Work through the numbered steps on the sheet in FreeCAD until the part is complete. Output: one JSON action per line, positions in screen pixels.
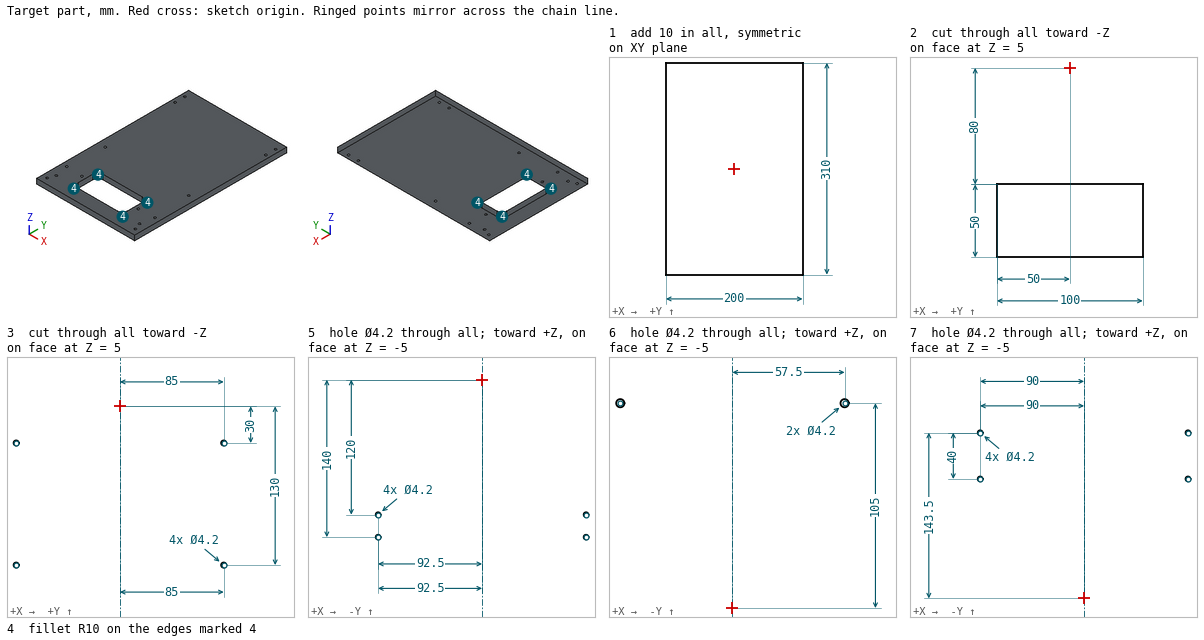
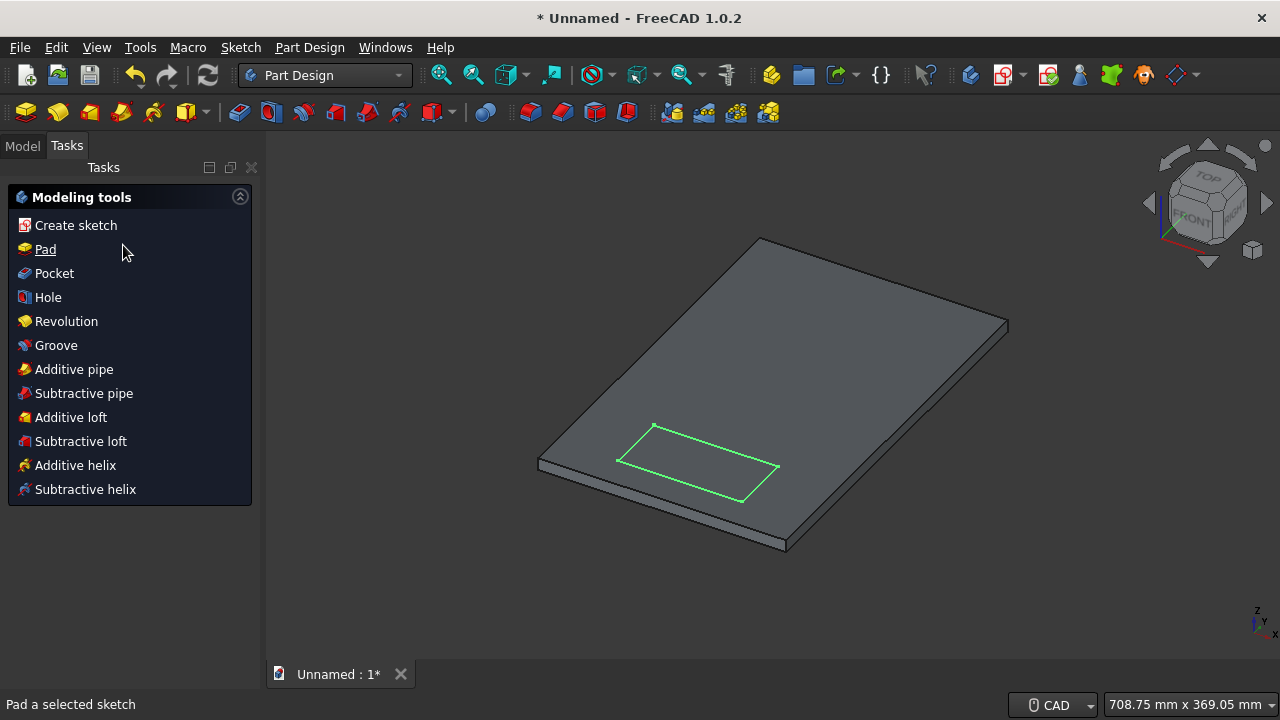
{"action": "left_click", "coordinate": [240, 112]}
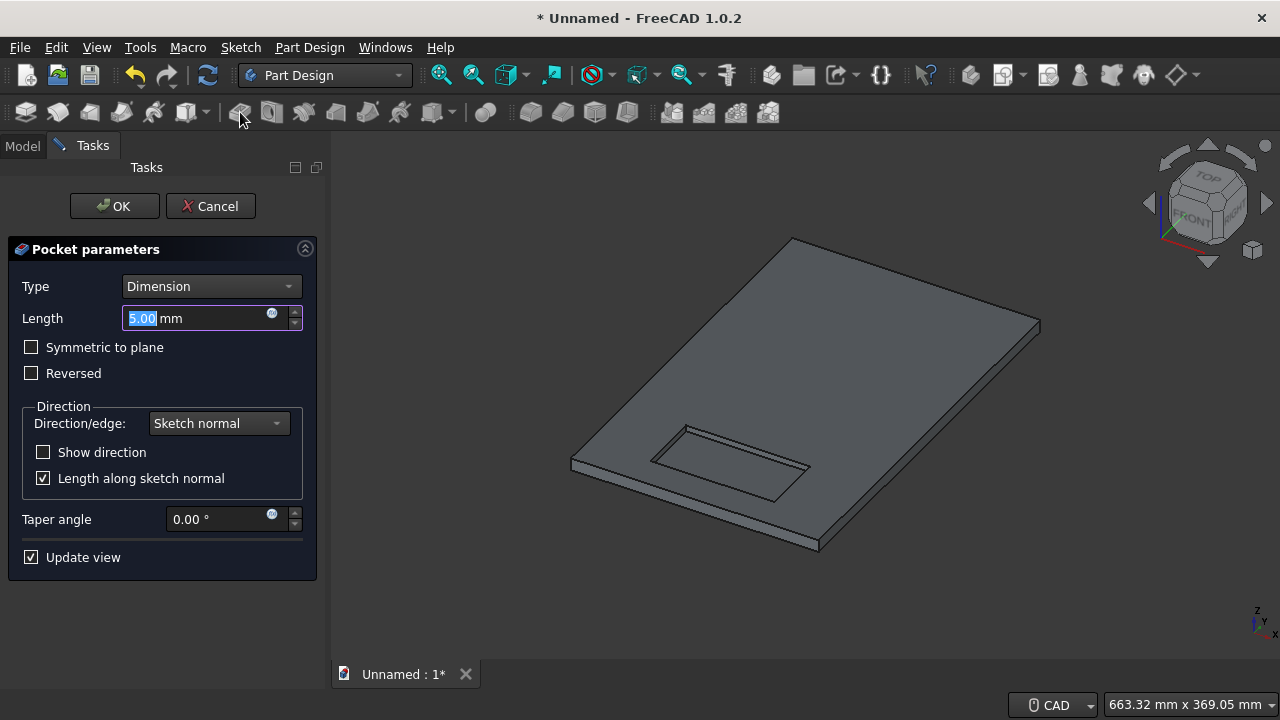
{"action": "left_click", "coordinate": [212, 286]}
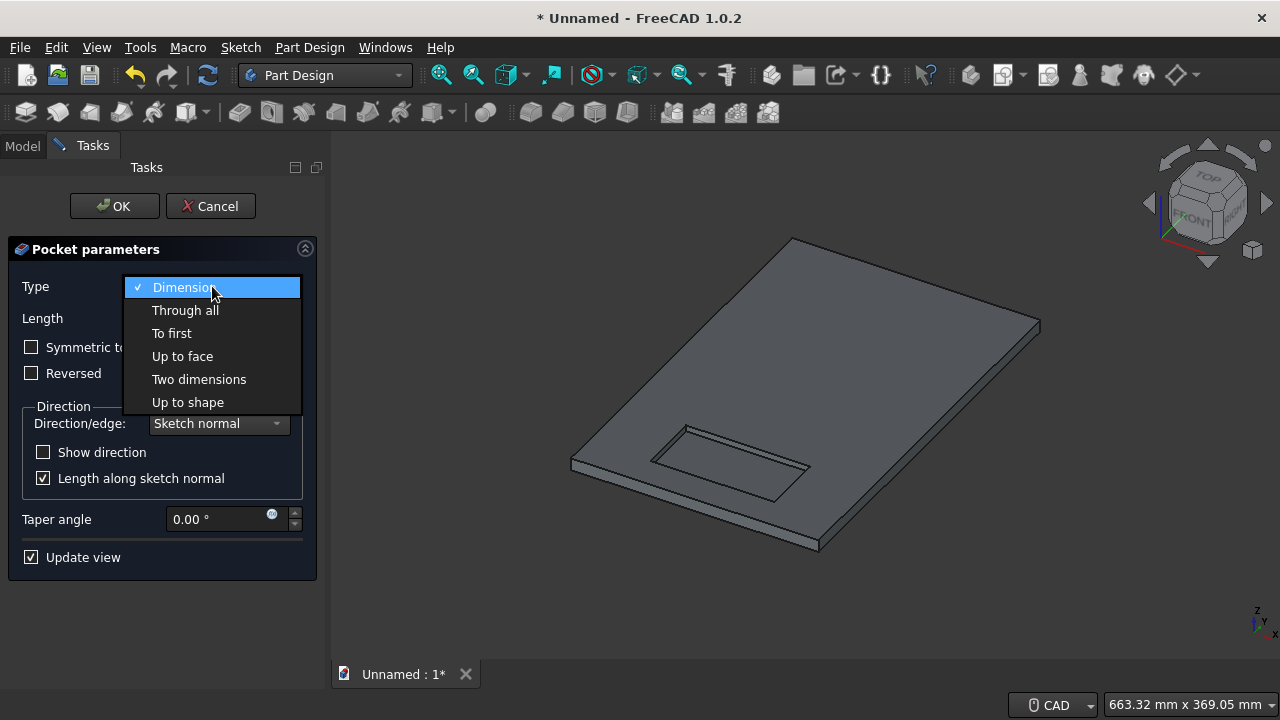
{"action": "left_click", "coordinate": [212, 310]}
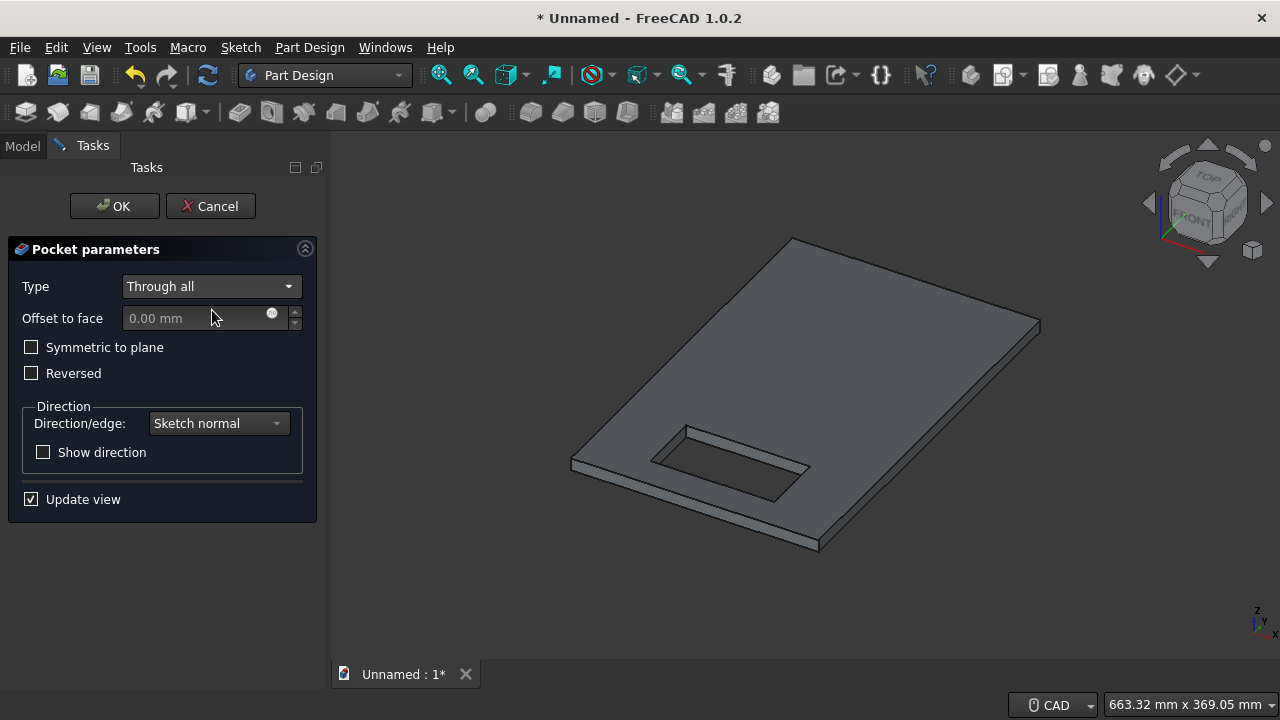
{"action": "left_click", "coordinate": [115, 206]}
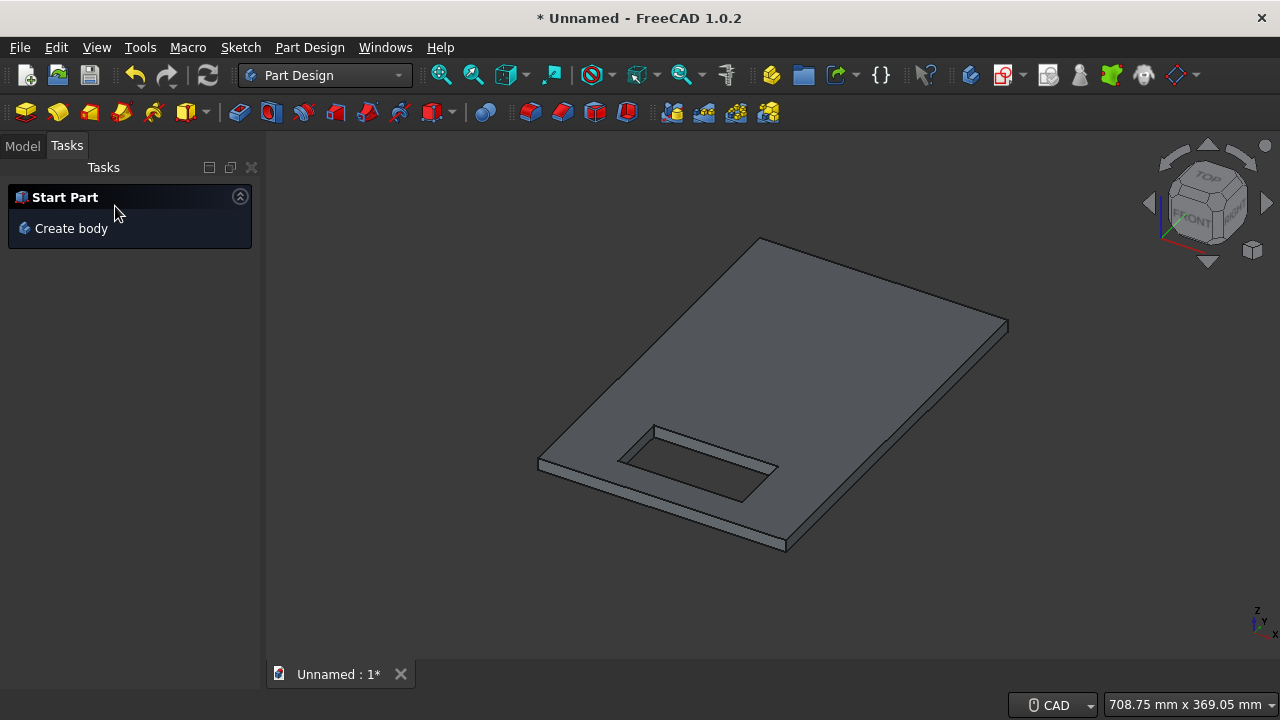
{"action": "left_click", "coordinate": [805, 357]}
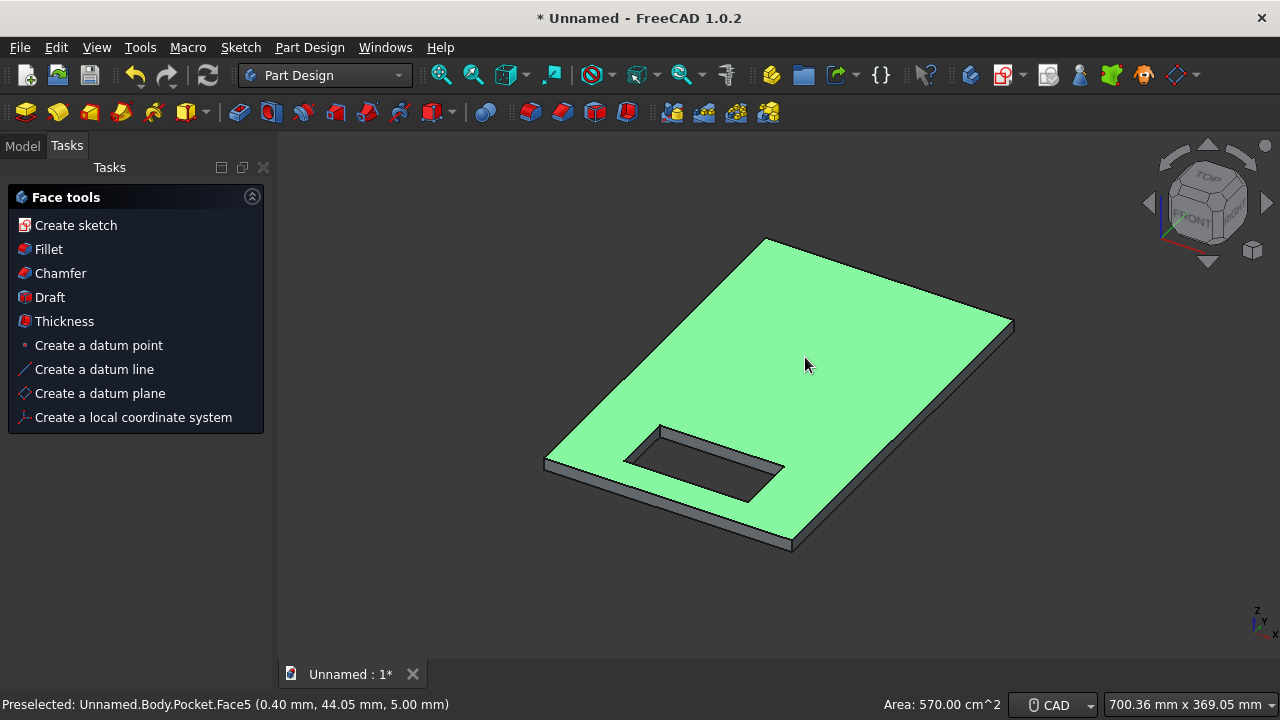
{"action": "left_click", "coordinate": [1004, 76]}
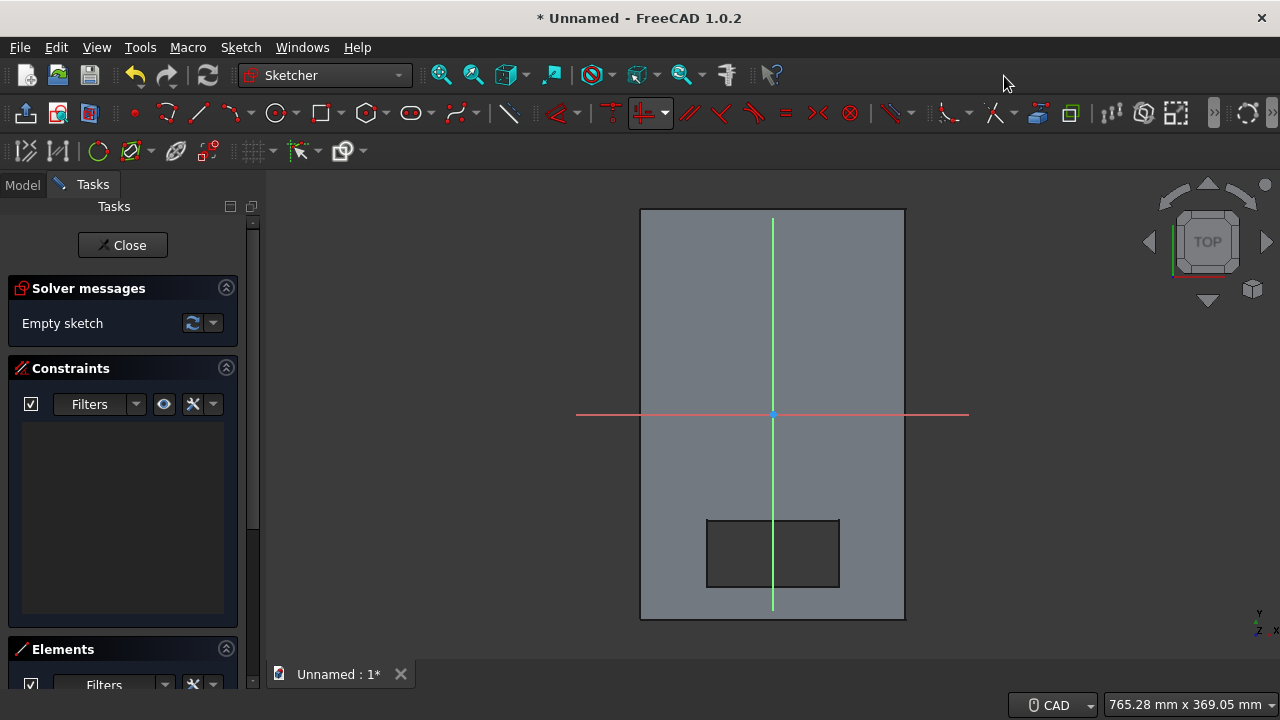
{"action": "scroll", "coordinate": [856, 608], "scroll_direction": "up", "scroll_amount": 3}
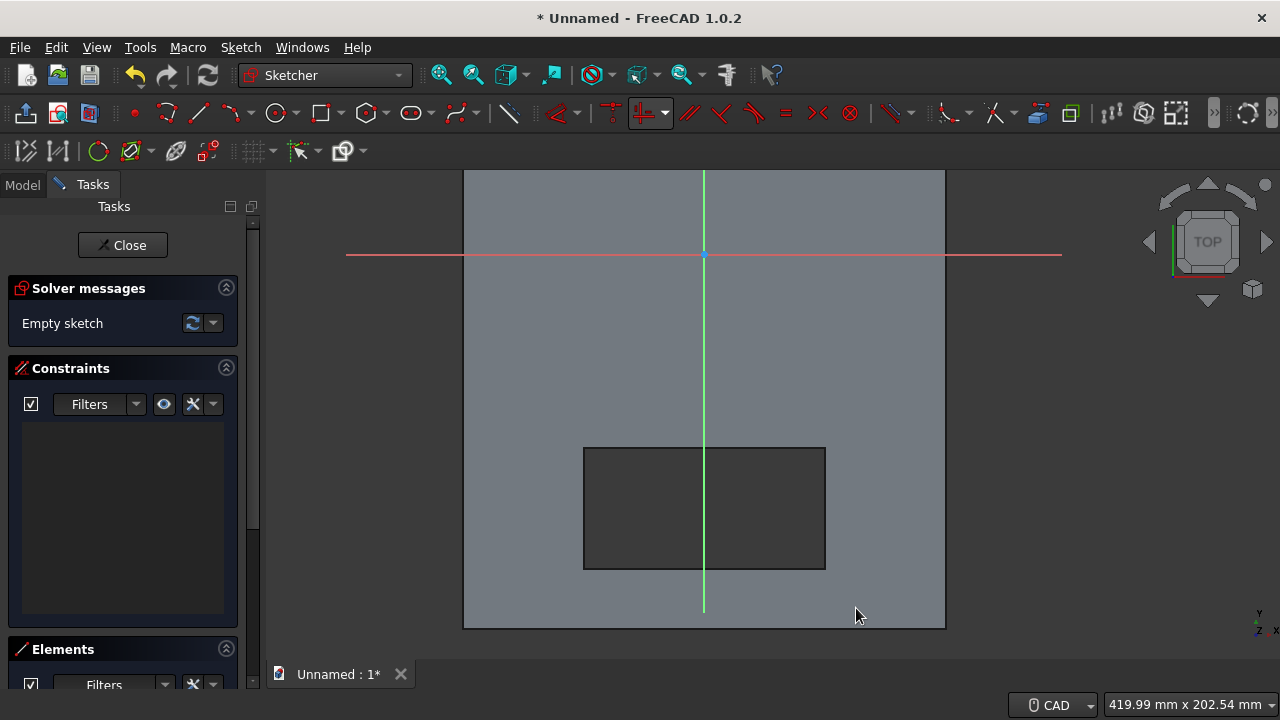
{"action": "key", "text": "g c"}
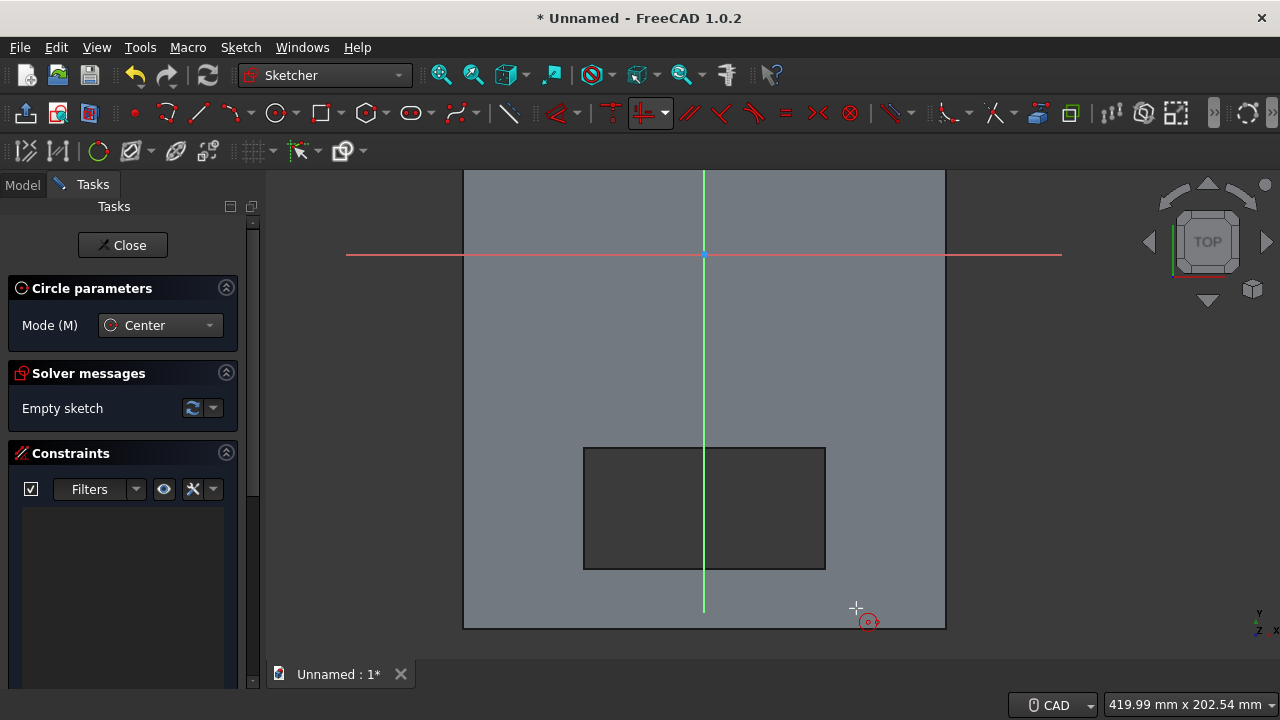
{"action": "scroll", "coordinate": [910, 569], "scroll_direction": "up", "scroll_amount": 8}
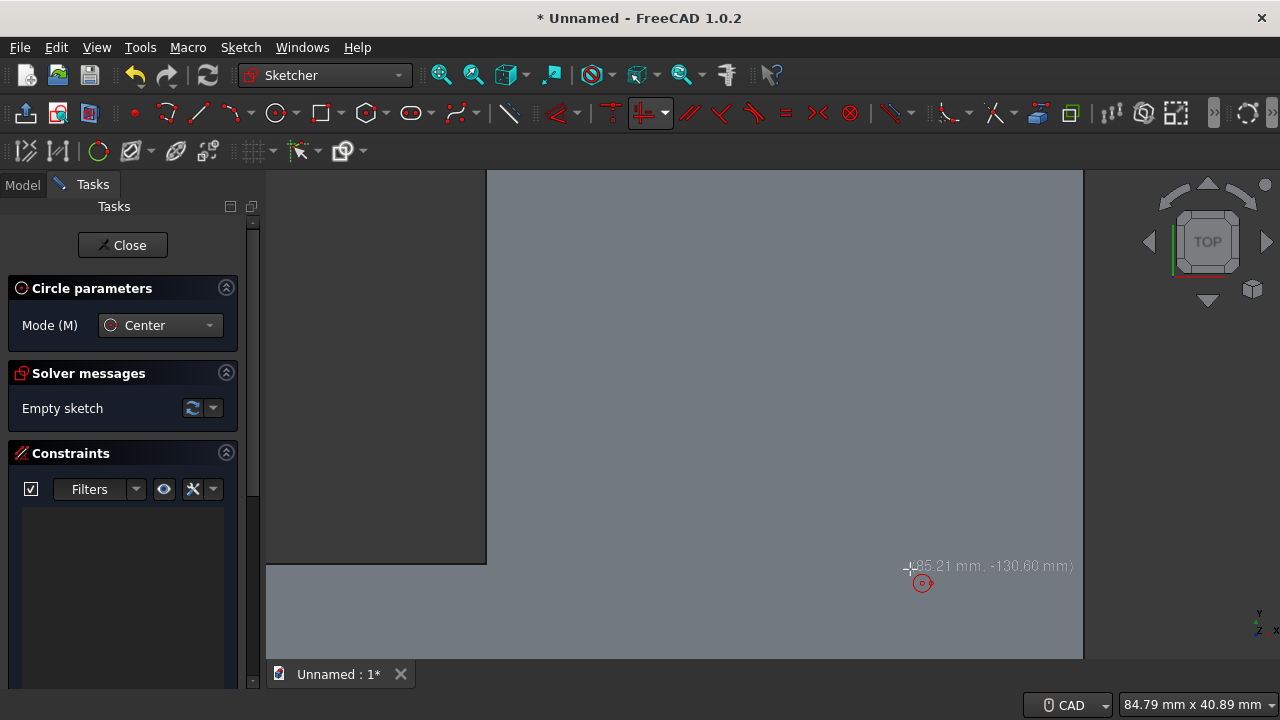
{"action": "scroll", "coordinate": [911, 570], "scroll_direction": "down", "scroll_amount": 8}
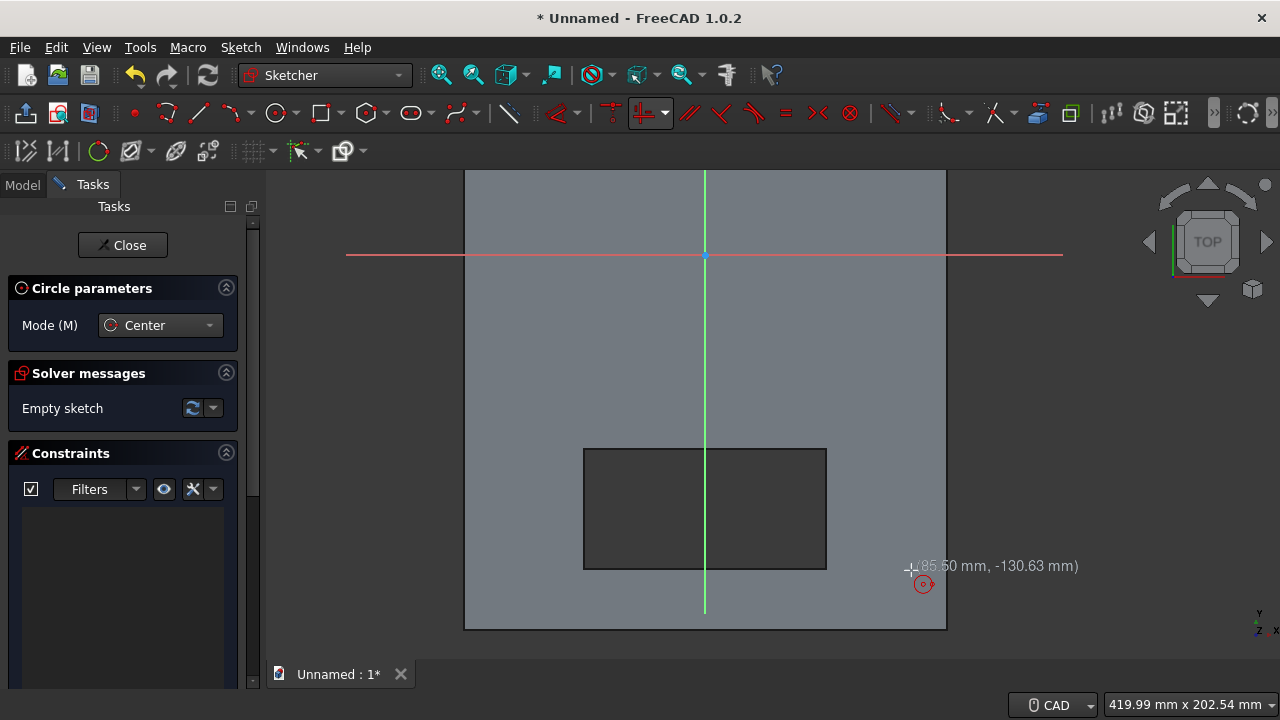
{"action": "left_click", "coordinate": [910, 569]}